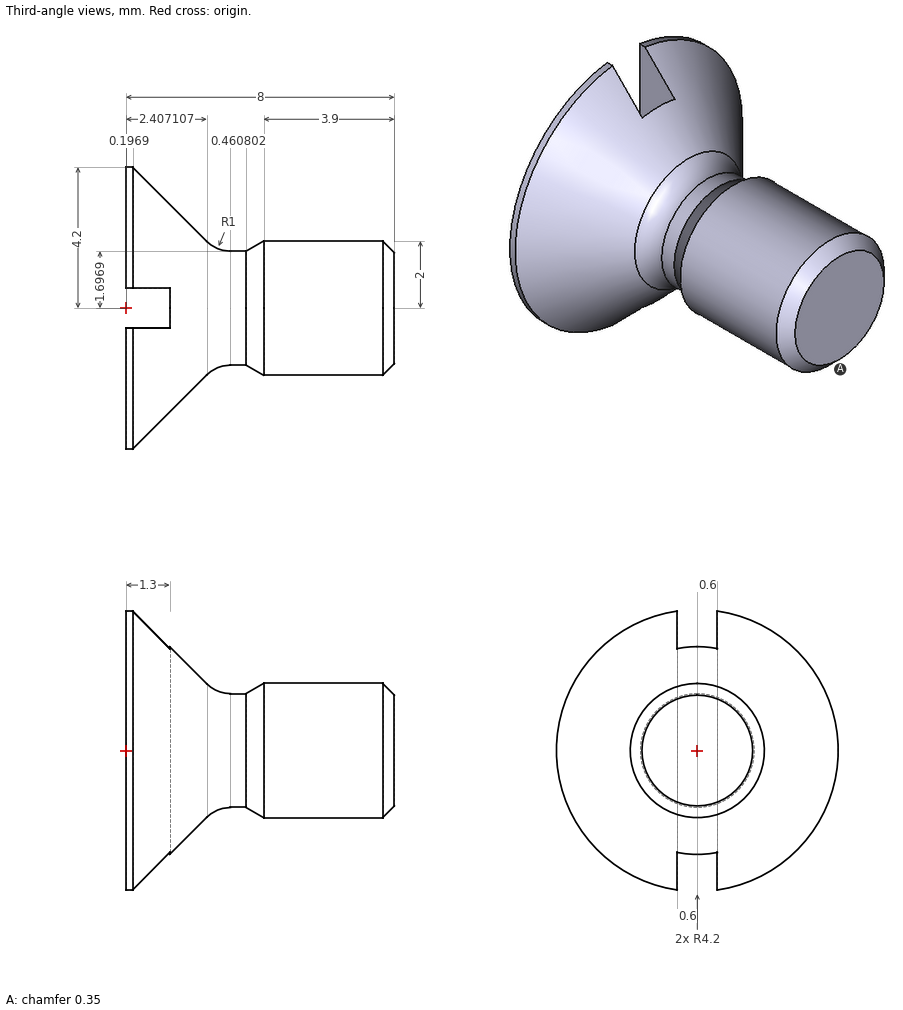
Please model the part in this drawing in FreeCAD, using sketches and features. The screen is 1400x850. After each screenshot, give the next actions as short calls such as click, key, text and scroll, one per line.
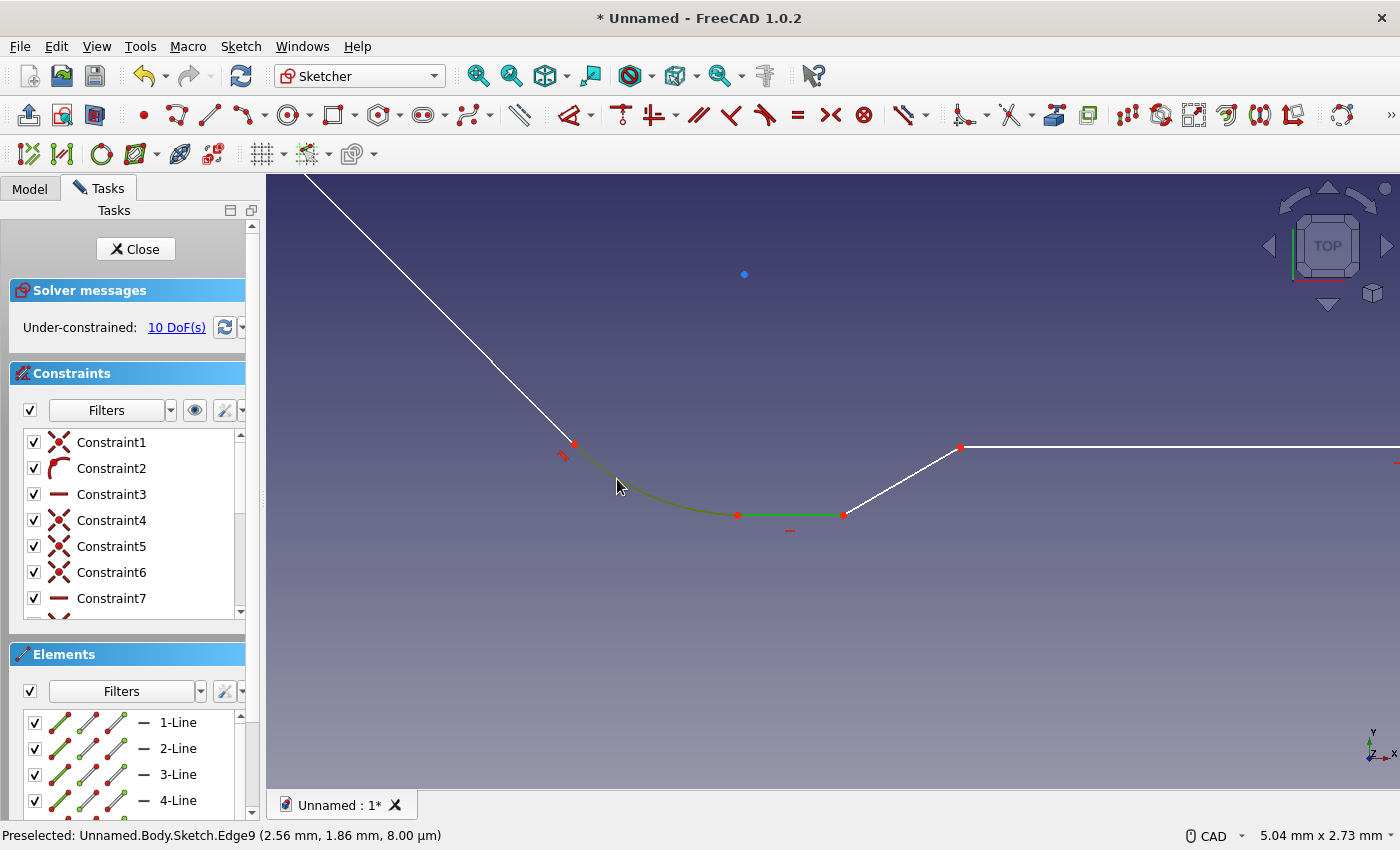
key(t)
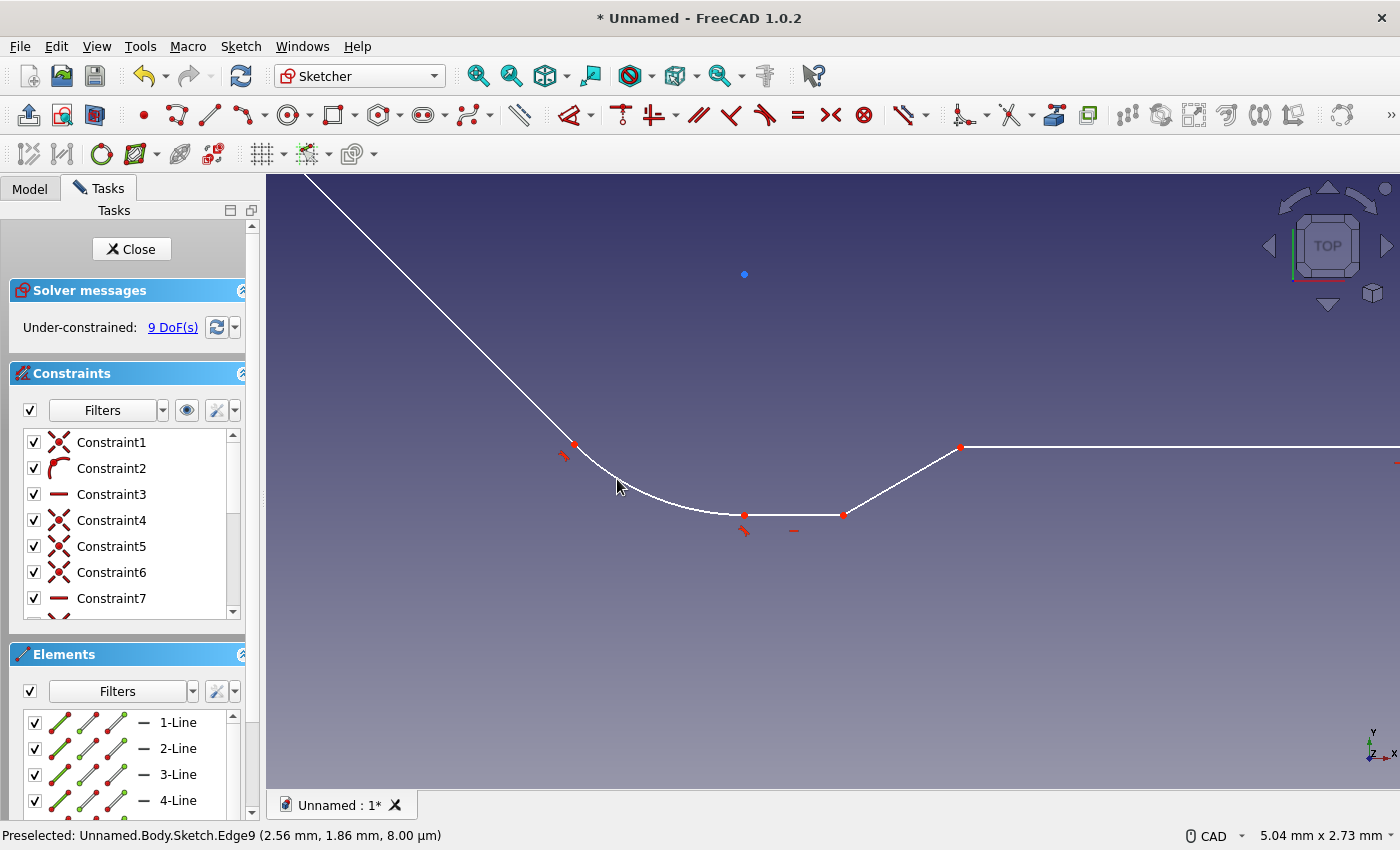
click(568, 116)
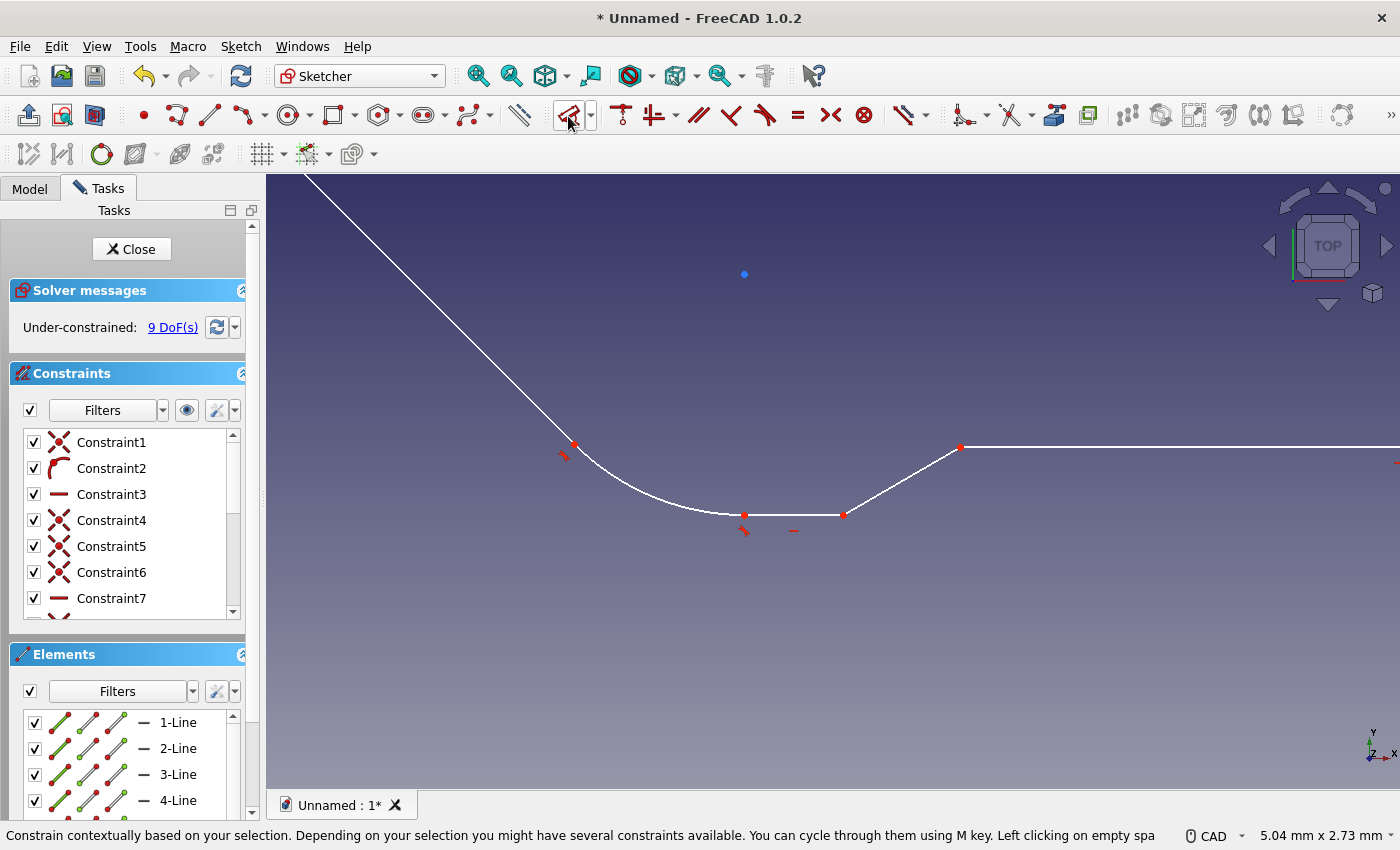
click(619, 480)
click(602, 507)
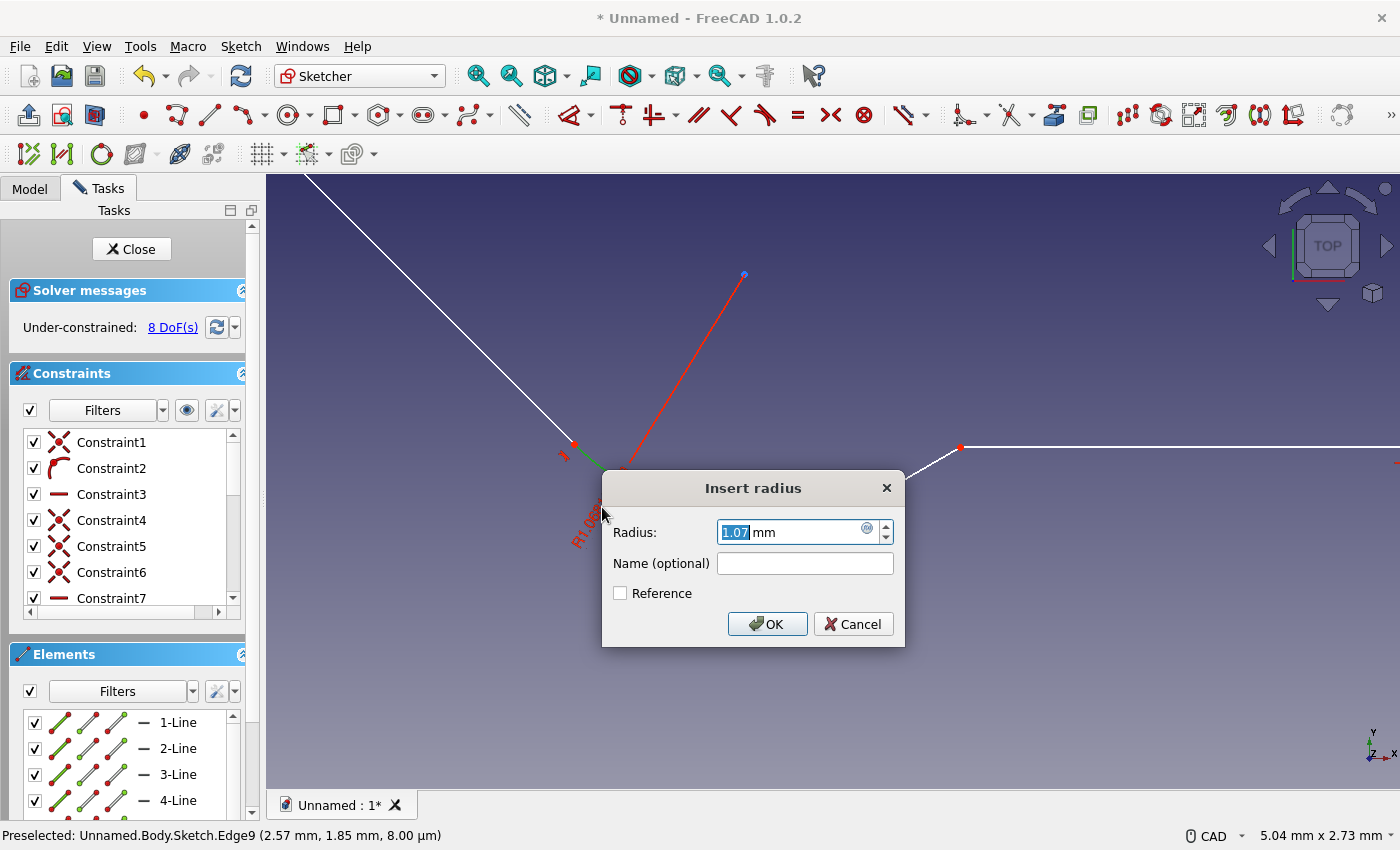
text(1)
key(Return)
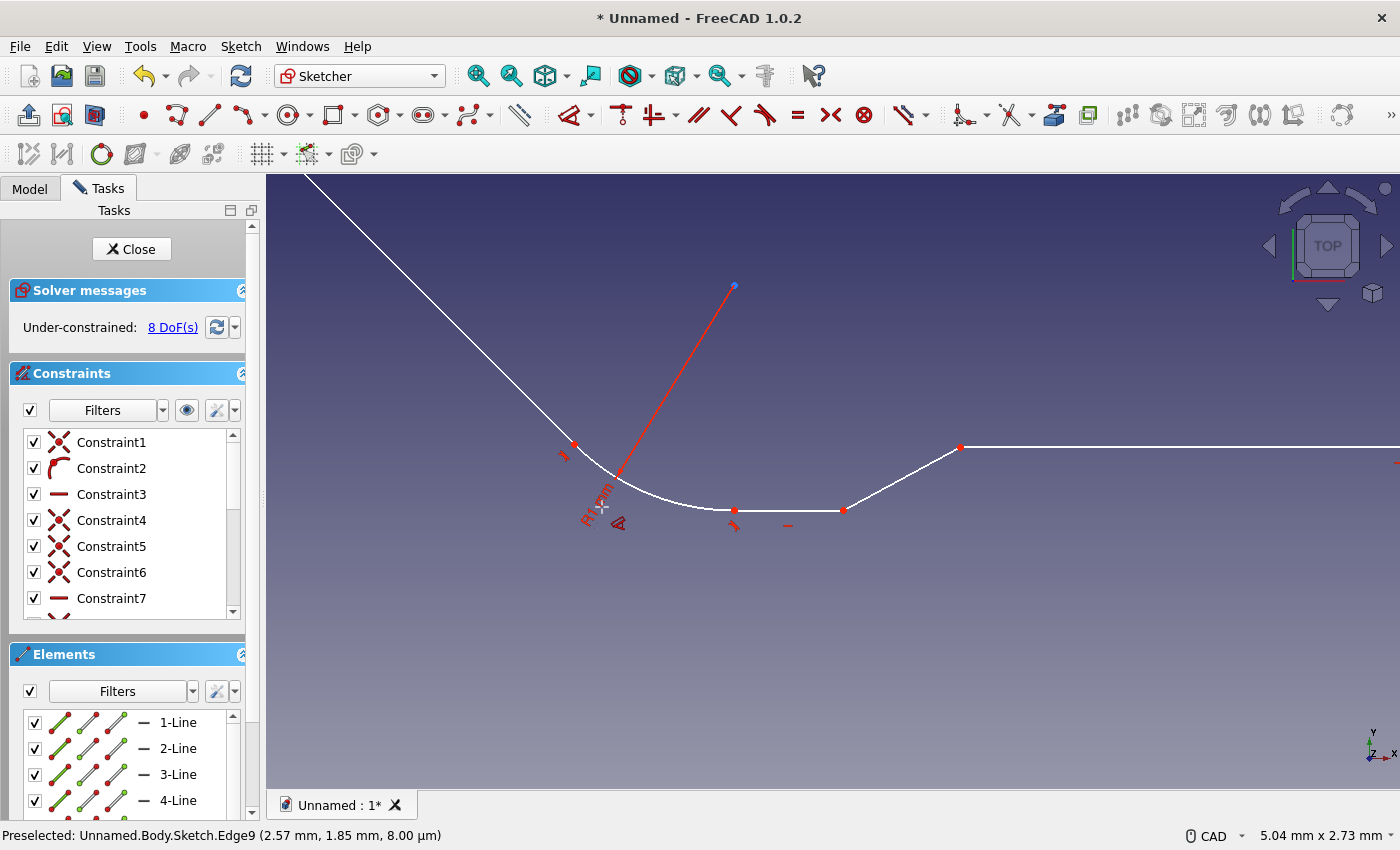
scroll(663, 516, down, 5)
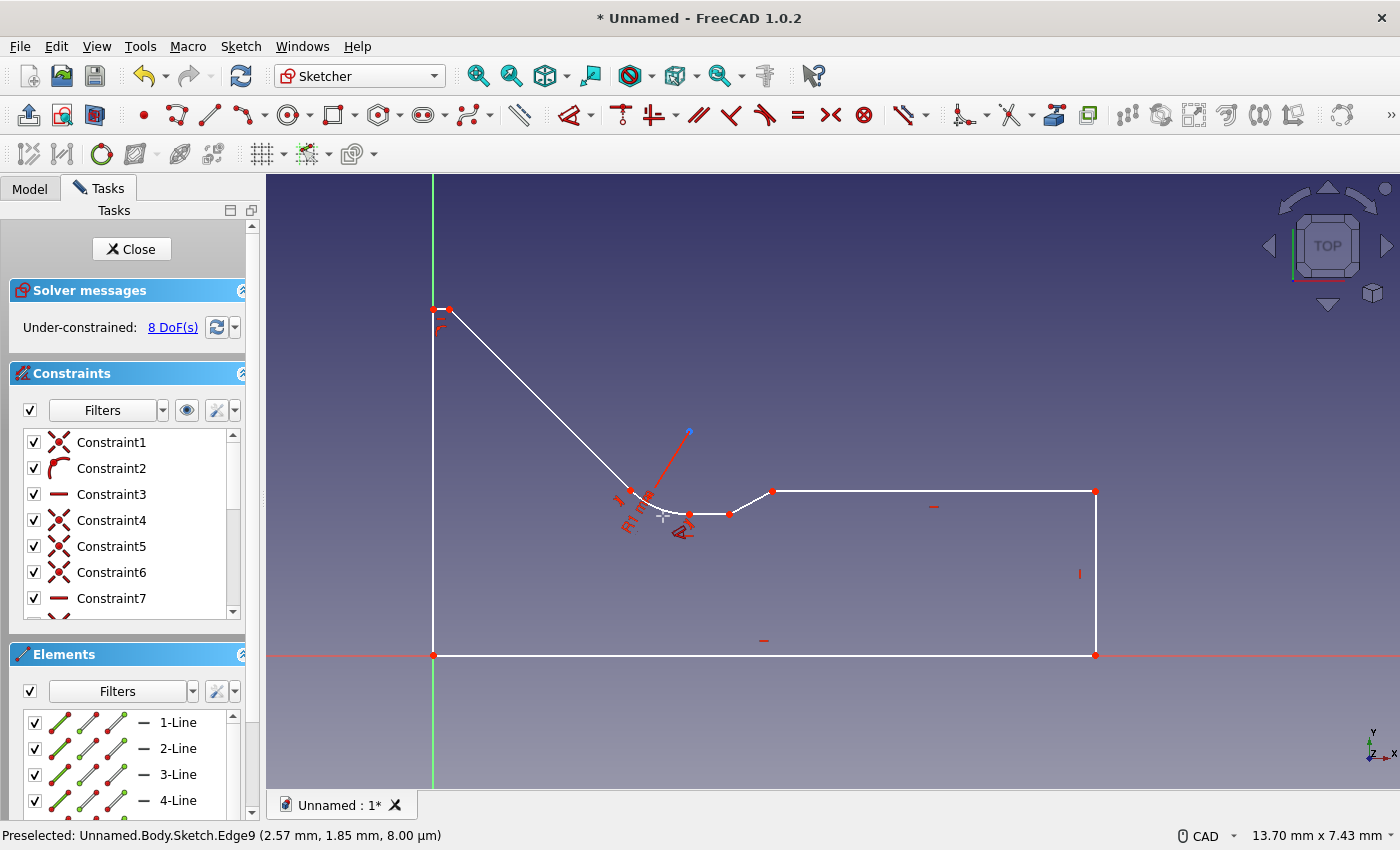
click(632, 656)
click(764, 690)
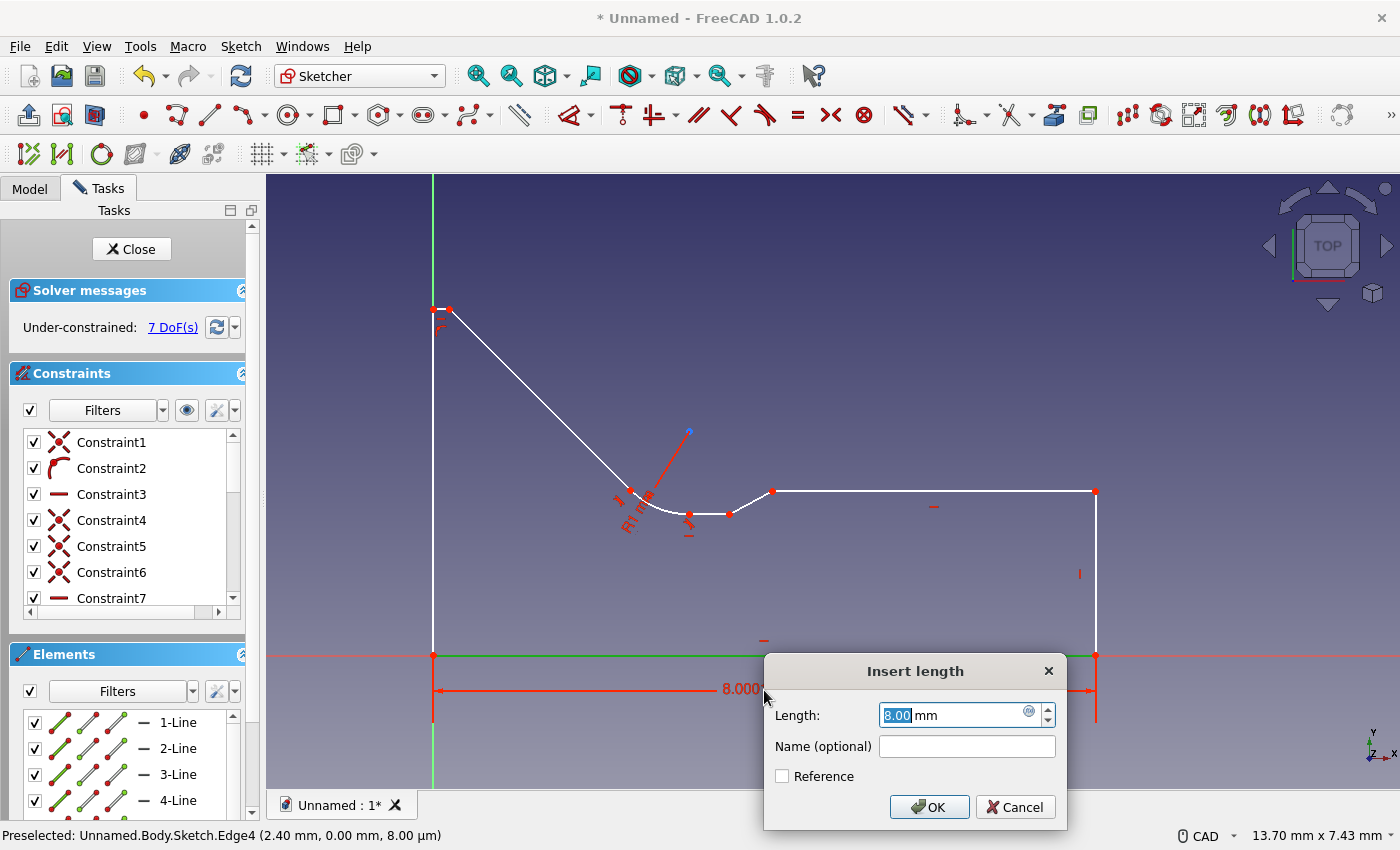
text(8)
key(Return)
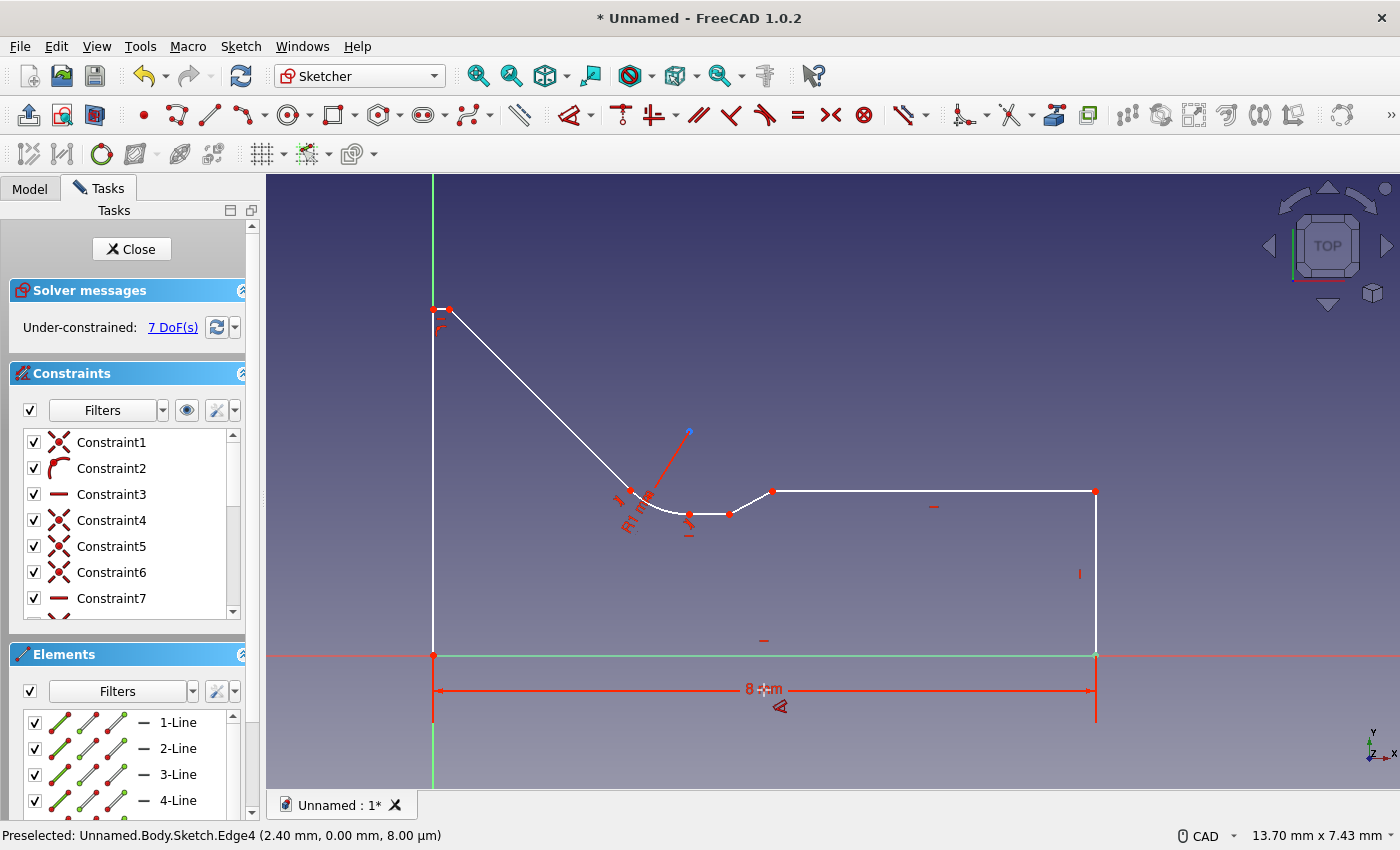
click(1096, 606)
click(1130, 573)